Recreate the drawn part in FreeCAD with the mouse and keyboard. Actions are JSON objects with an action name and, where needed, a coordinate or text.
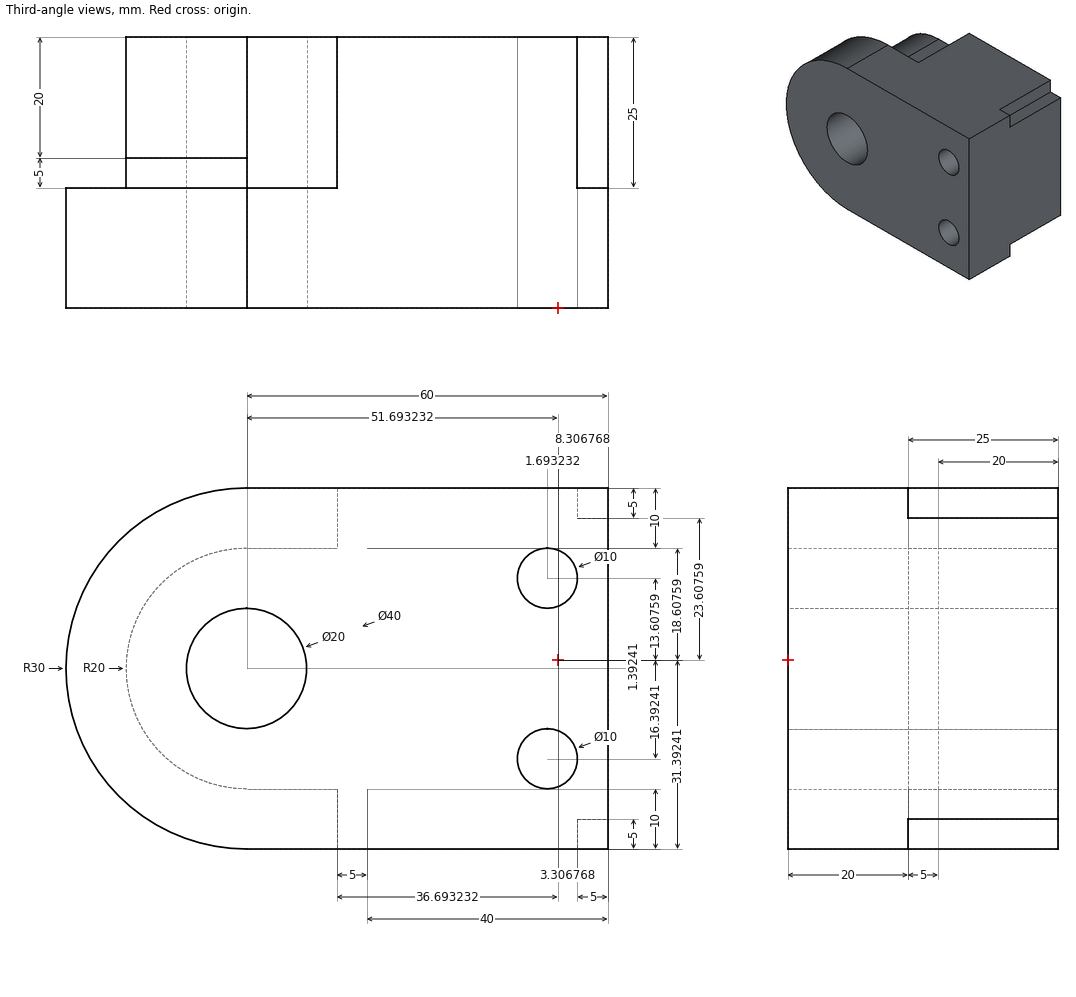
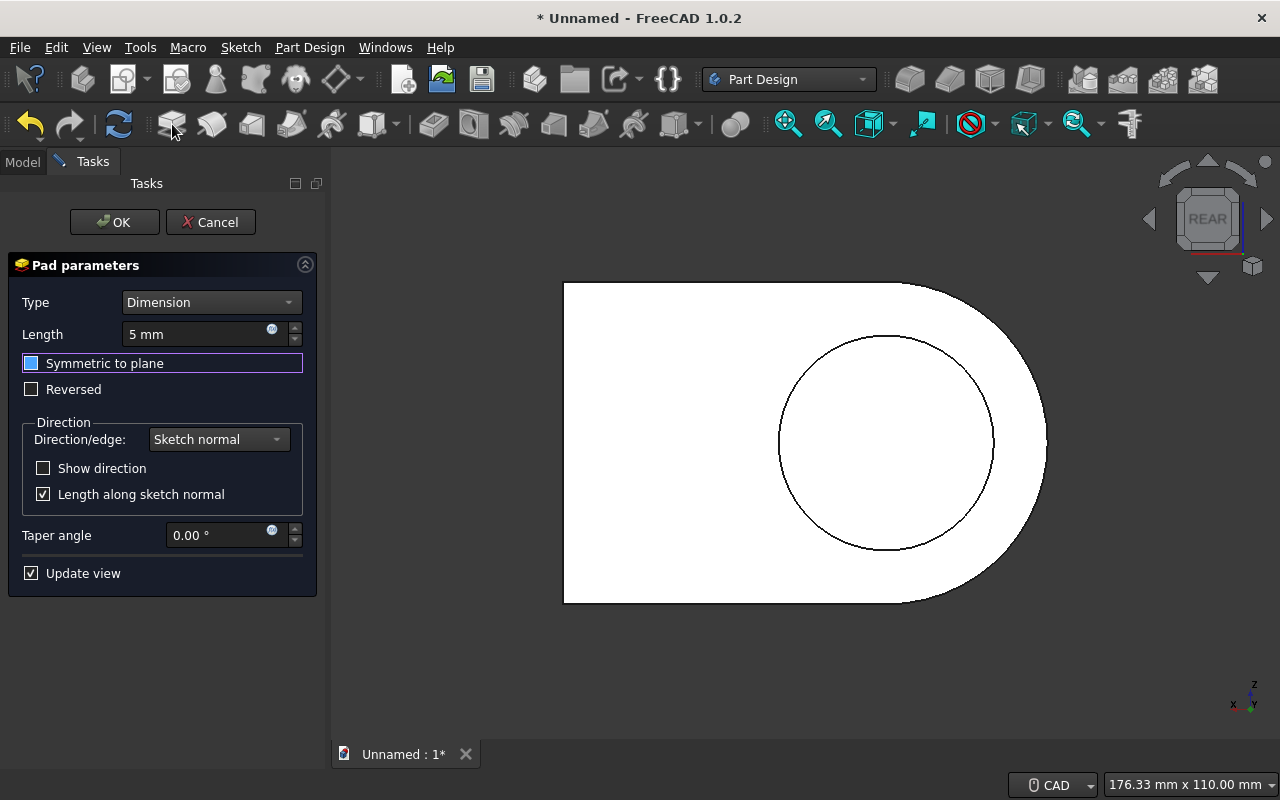
{"action": "left_click", "coordinate": [115, 222]}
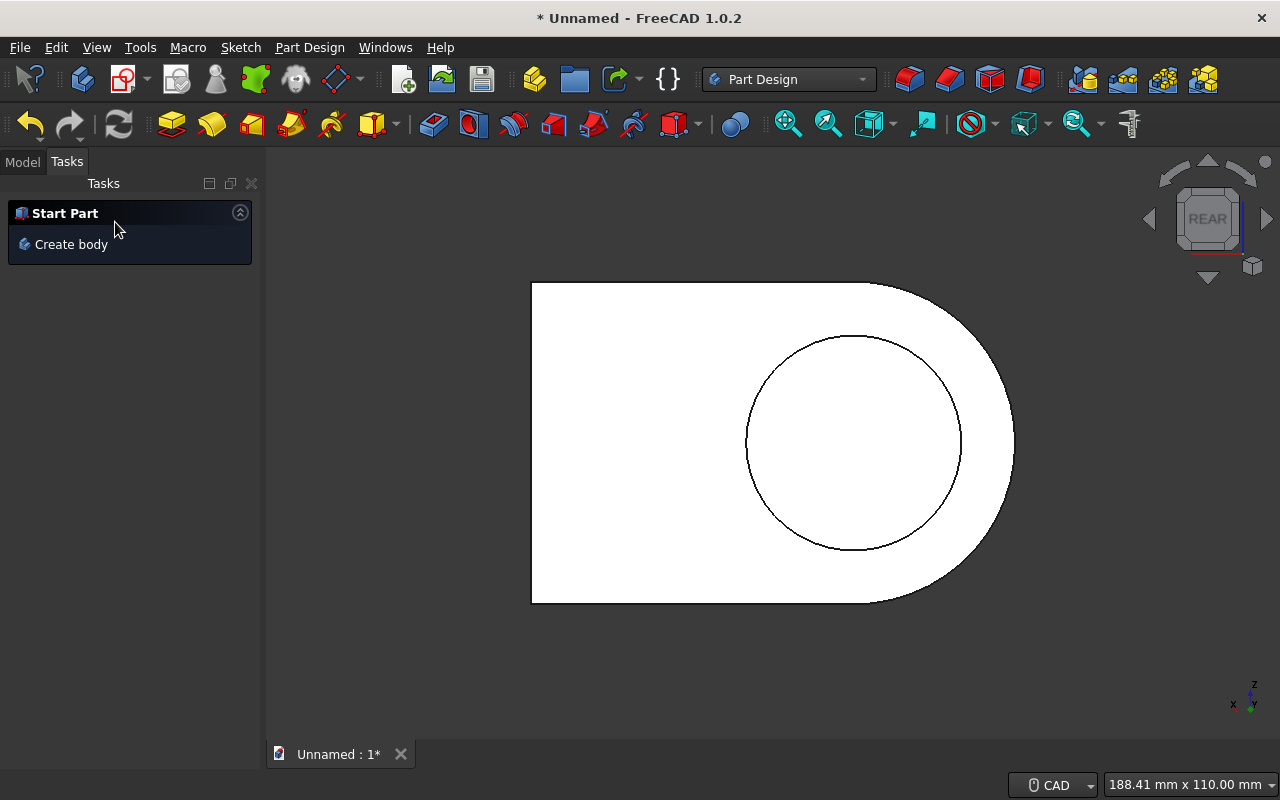
{"action": "left_click", "coordinate": [635, 396]}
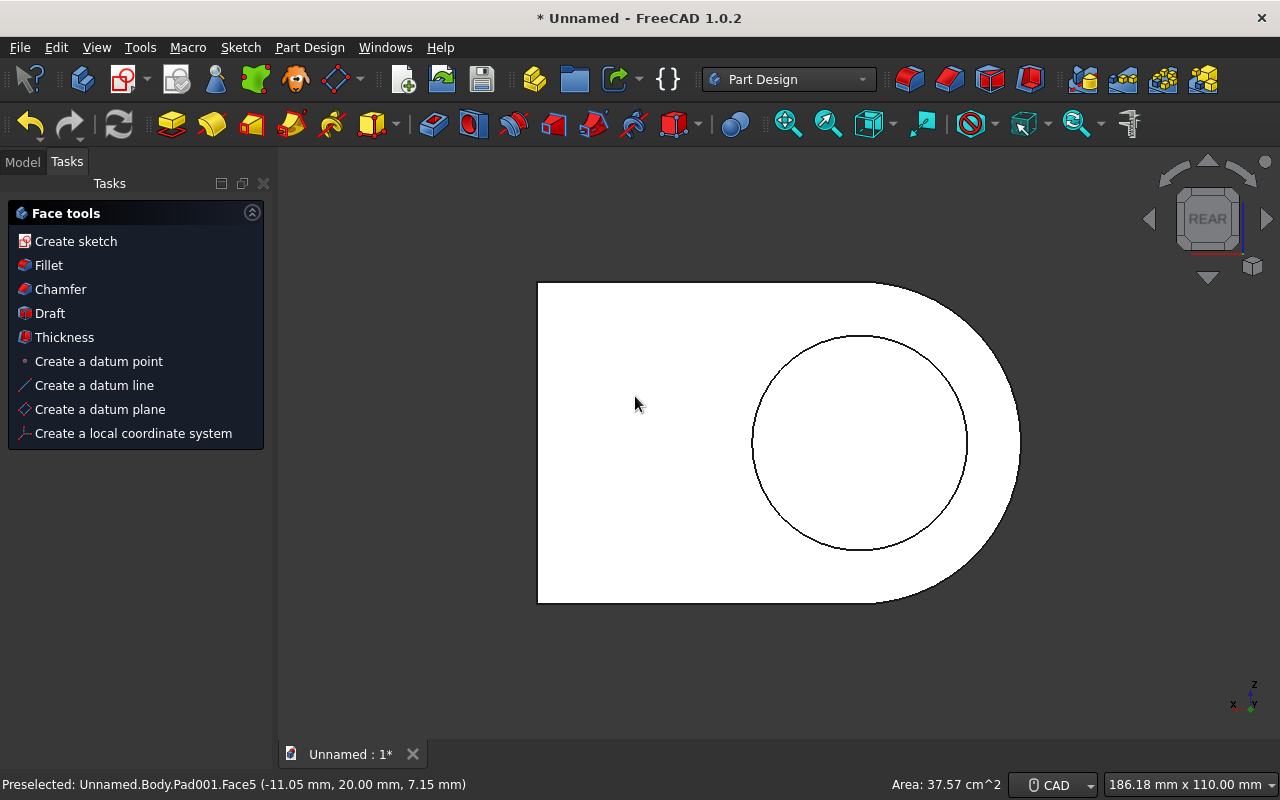
{"action": "left_click", "coordinate": [124, 80]}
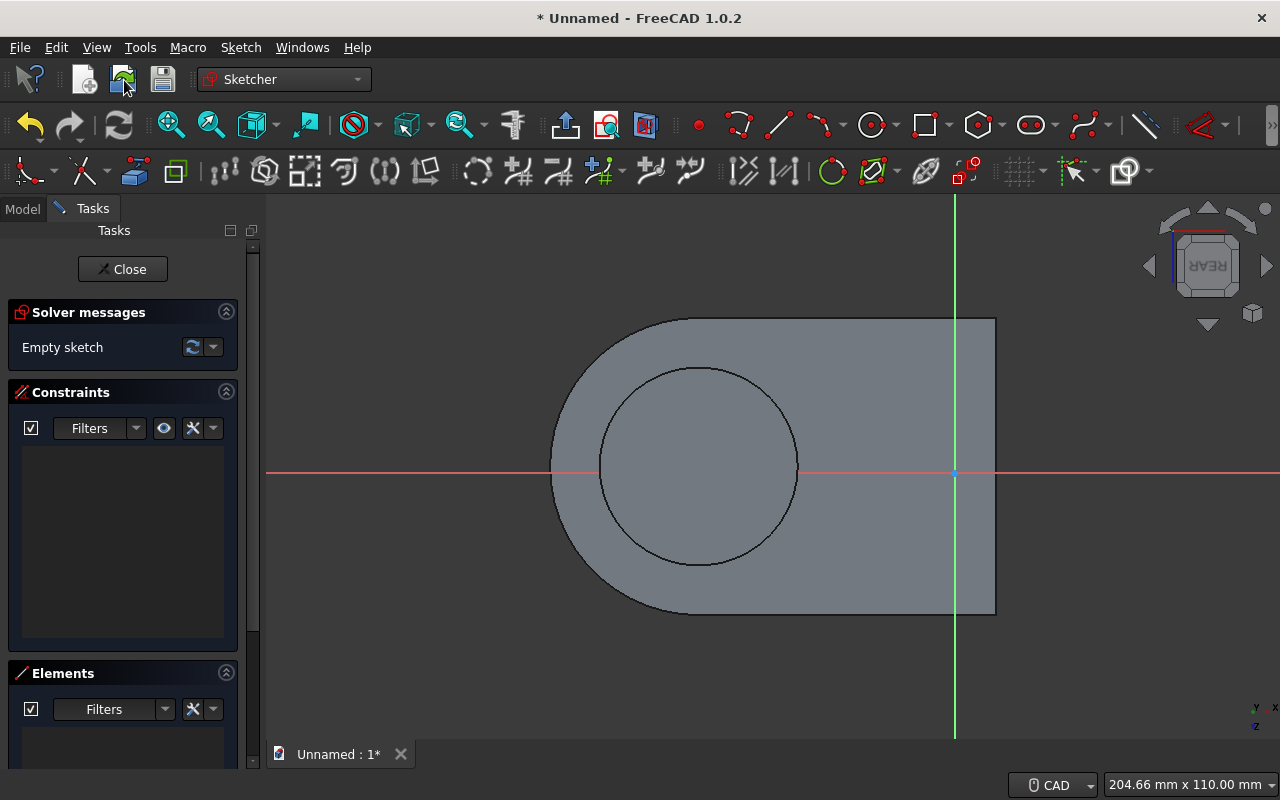
{"action": "left_click", "coordinate": [646, 126]}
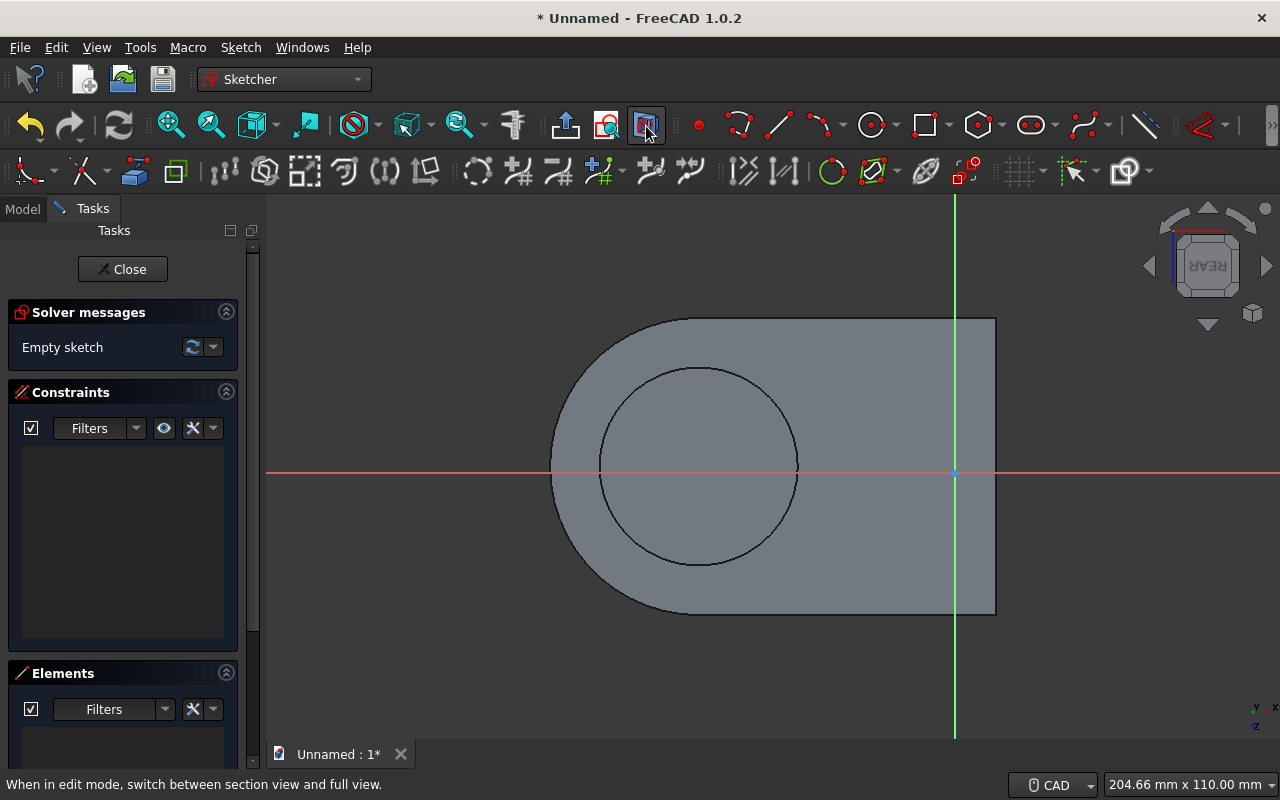
{"action": "scroll", "coordinate": [987, 466], "scroll_direction": "up", "scroll_amount": 2}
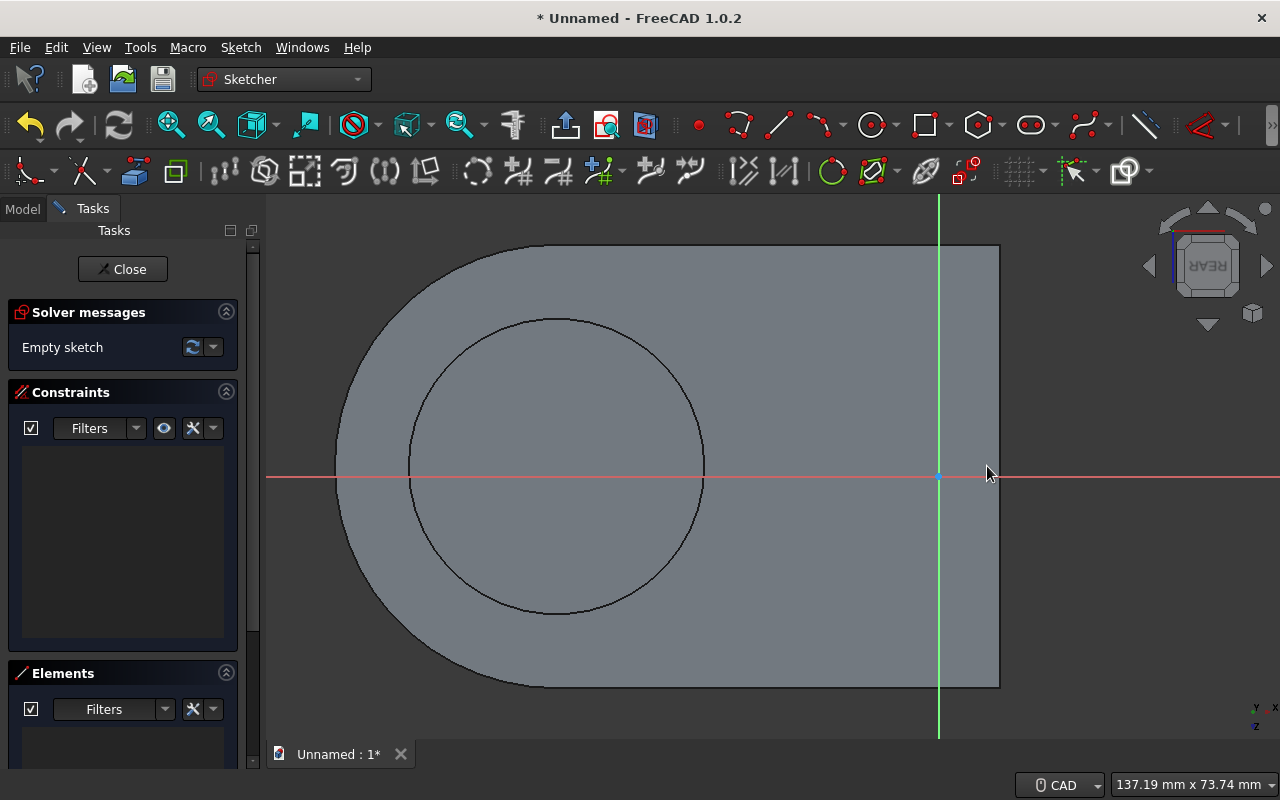
{"action": "key", "text": "g m"}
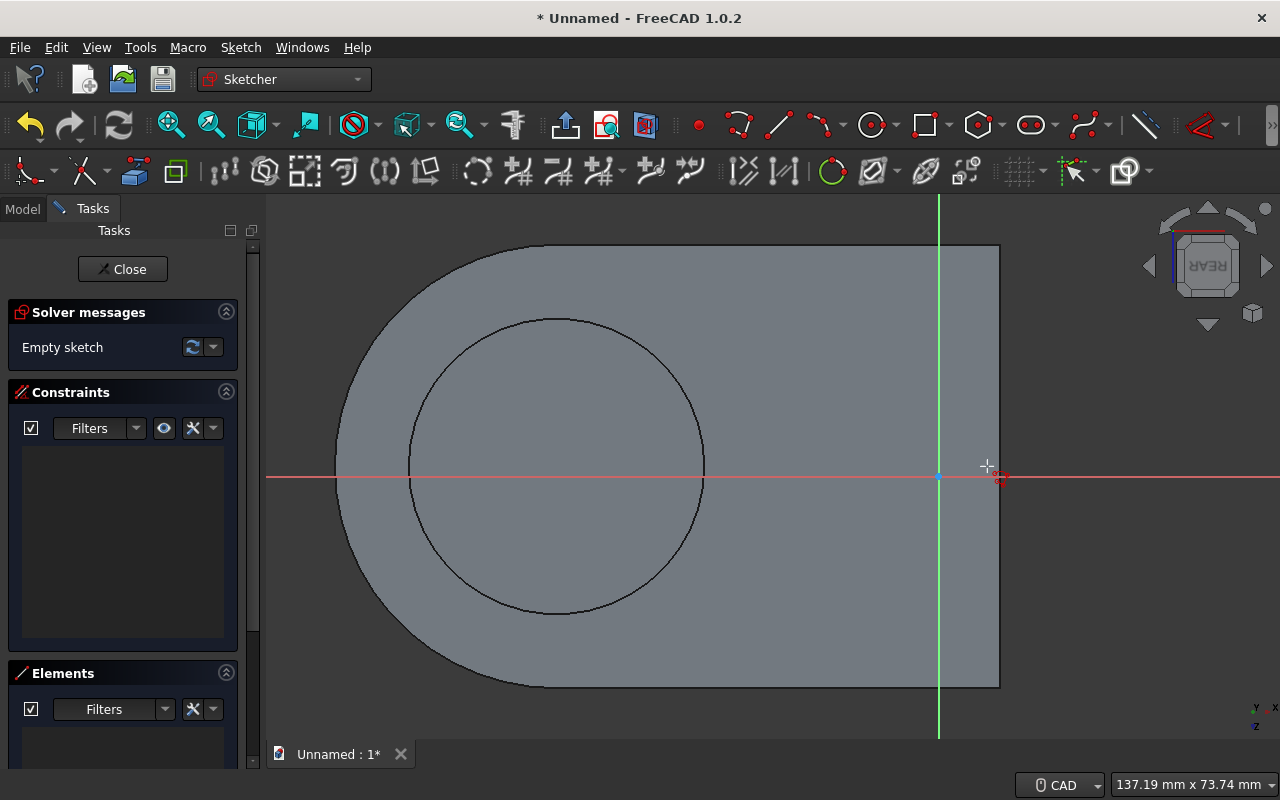
{"action": "left_click", "coordinate": [557, 614]}
{"action": "left_click", "coordinate": [1000, 614]}
{"action": "left_click", "coordinate": [1000, 319]}
{"action": "left_click", "coordinate": [557, 319]}
{"action": "right_click", "coordinate": [557, 319]}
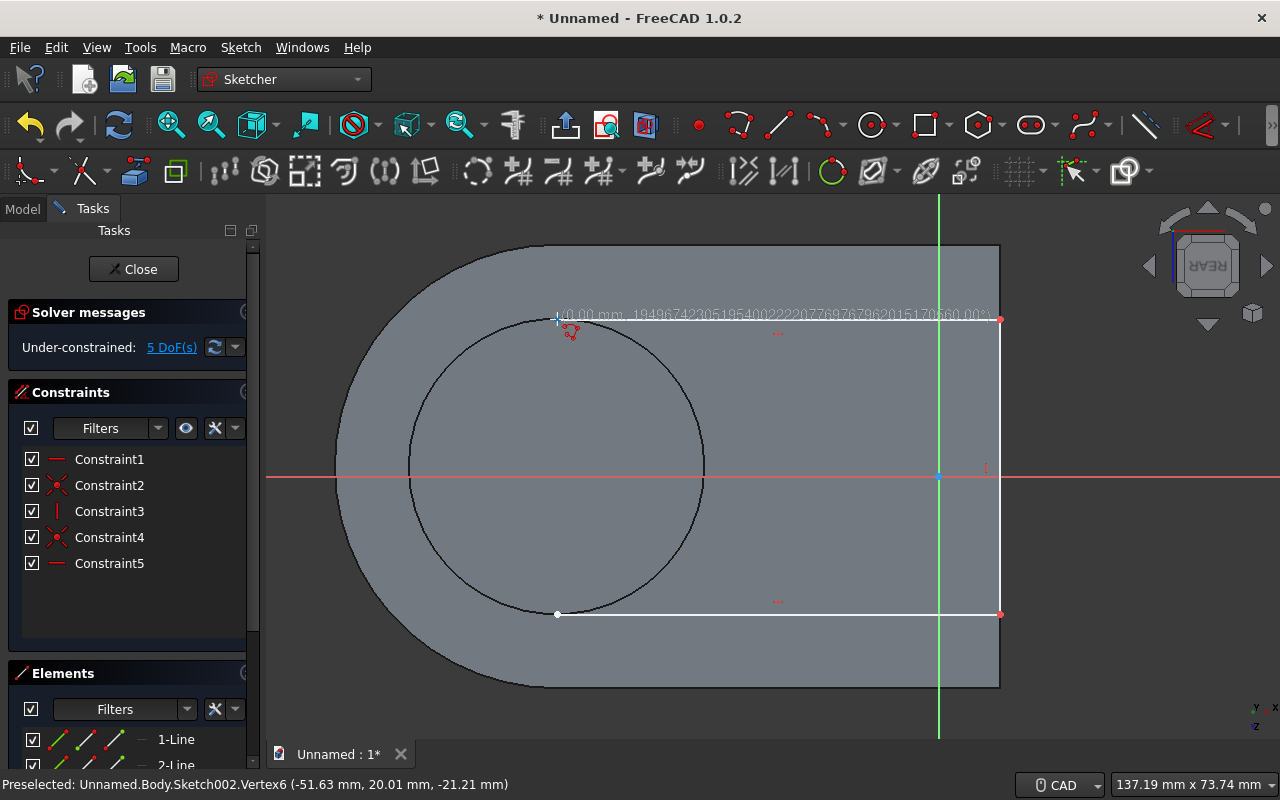
{"action": "left_click", "coordinate": [820, 126]}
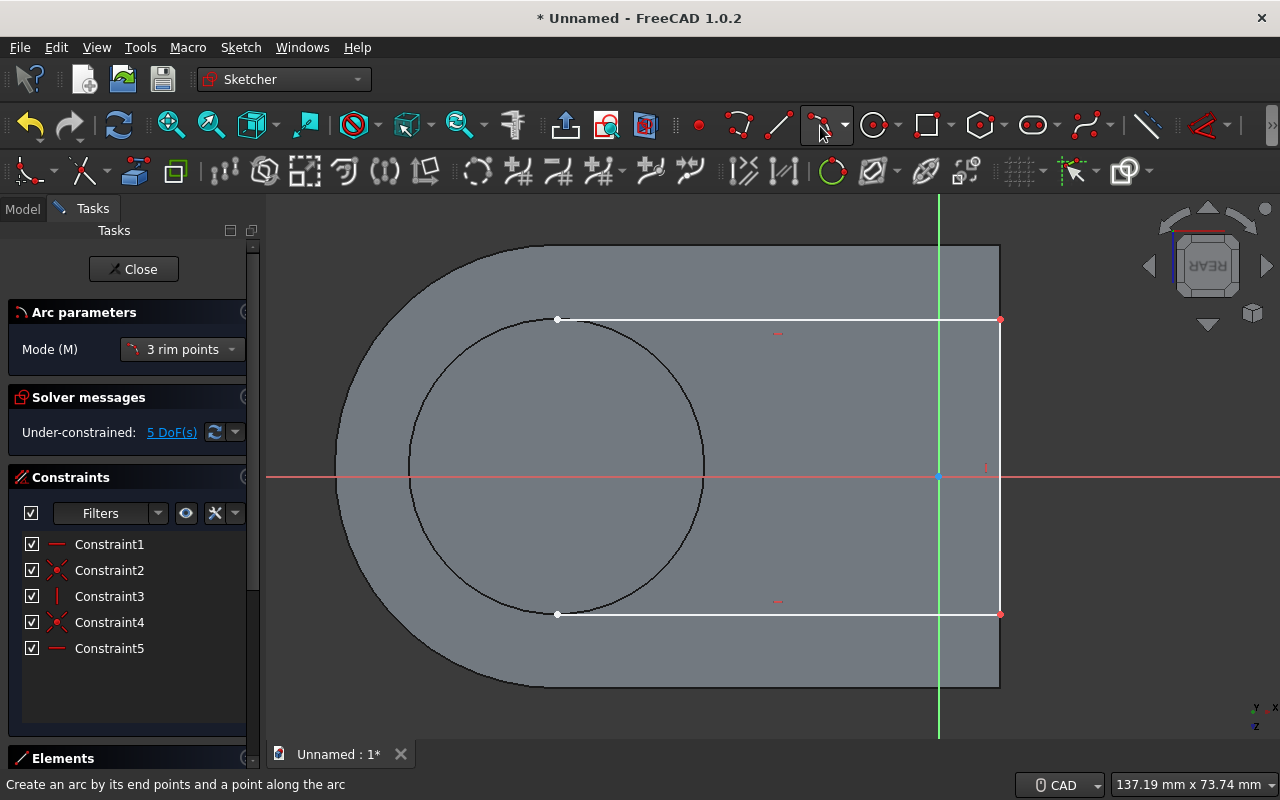
{"action": "left_click", "coordinate": [557, 320]}
{"action": "left_click", "coordinate": [557, 615]}
{"action": "left_click", "coordinate": [416, 421]}
{"action": "key", "text": "Escape"}